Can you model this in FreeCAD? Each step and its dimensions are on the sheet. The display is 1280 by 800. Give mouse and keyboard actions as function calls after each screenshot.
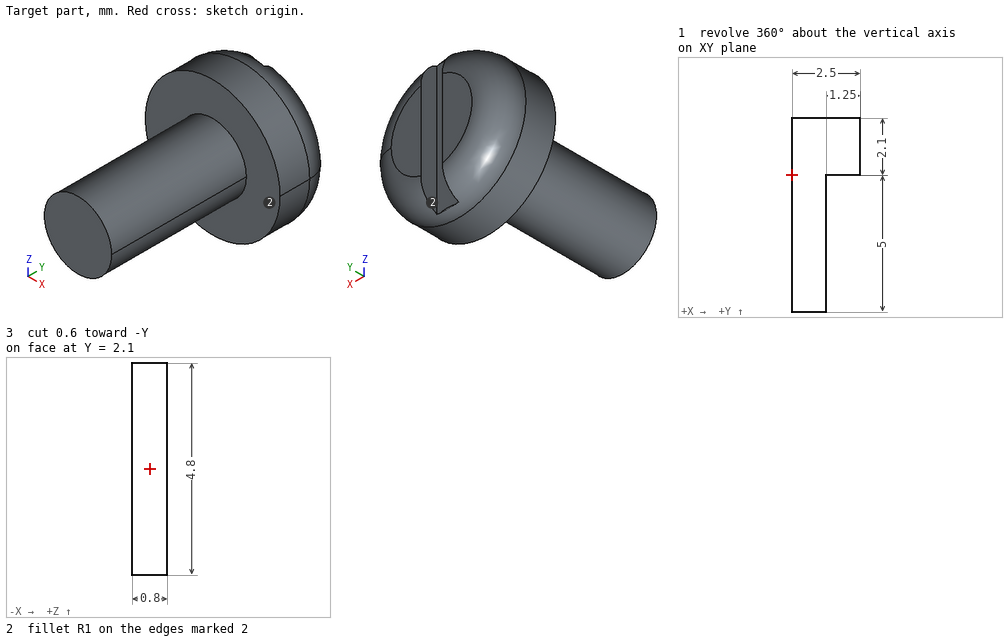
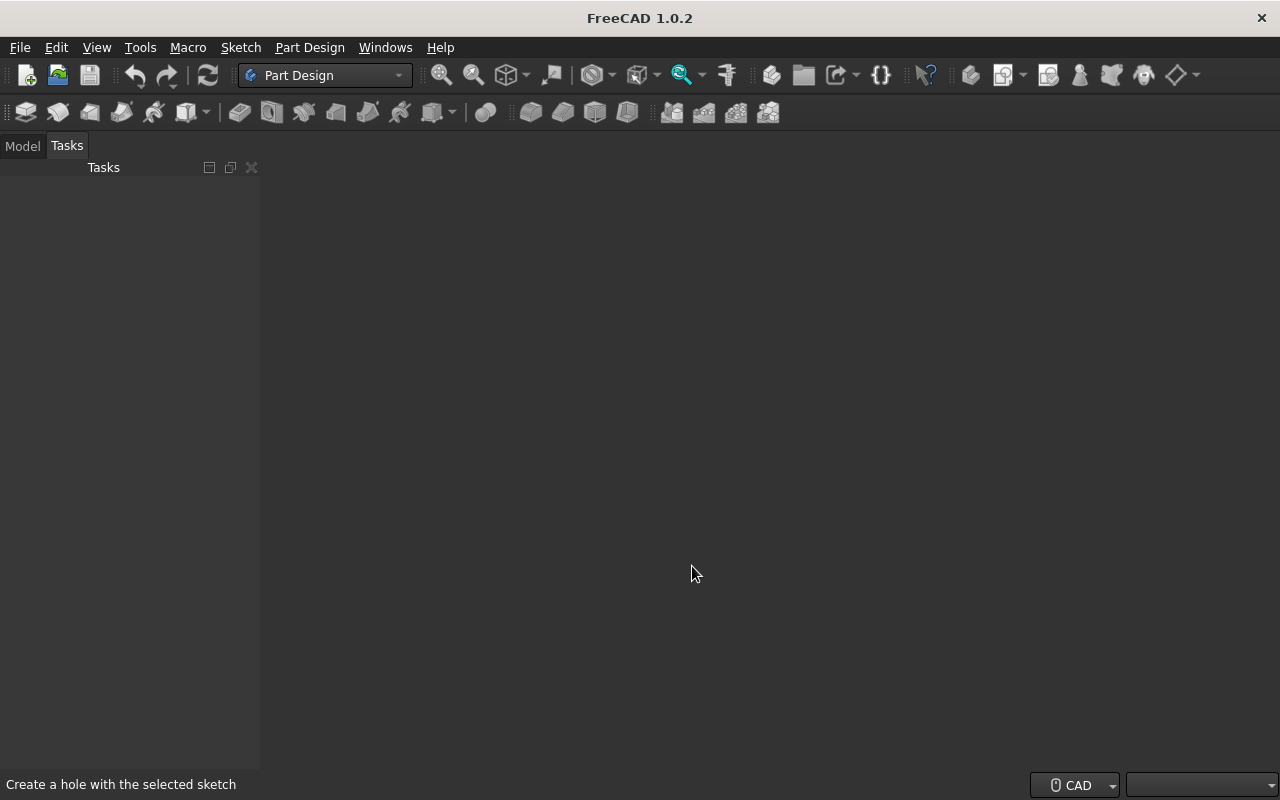
click(26, 76)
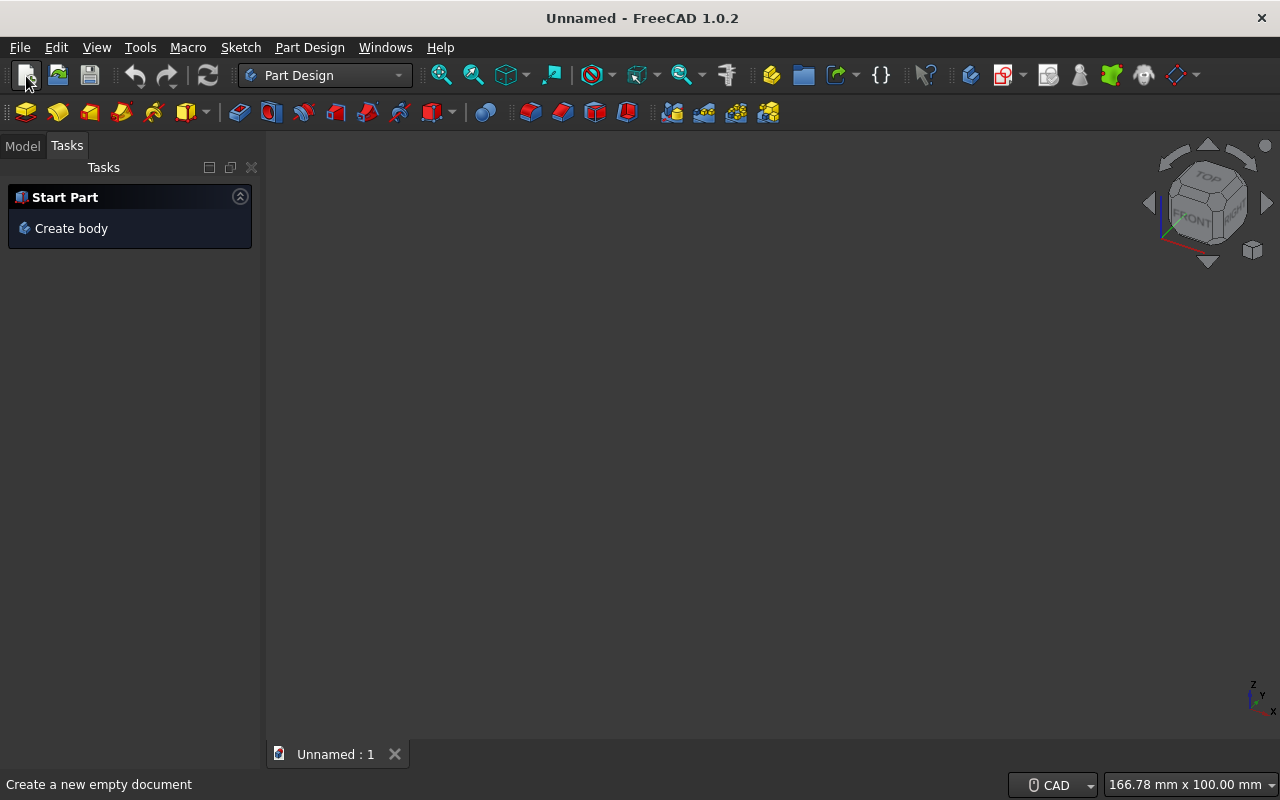
click(1004, 76)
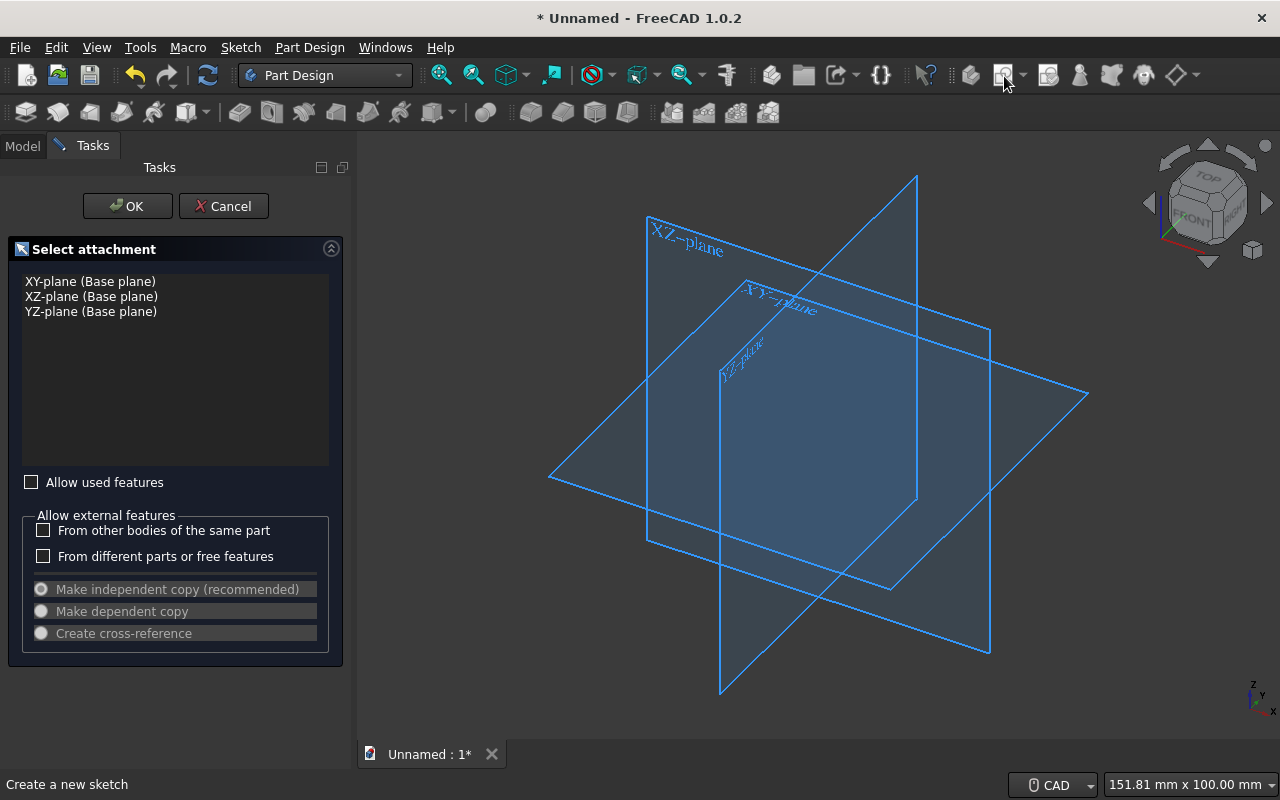
click(82, 282)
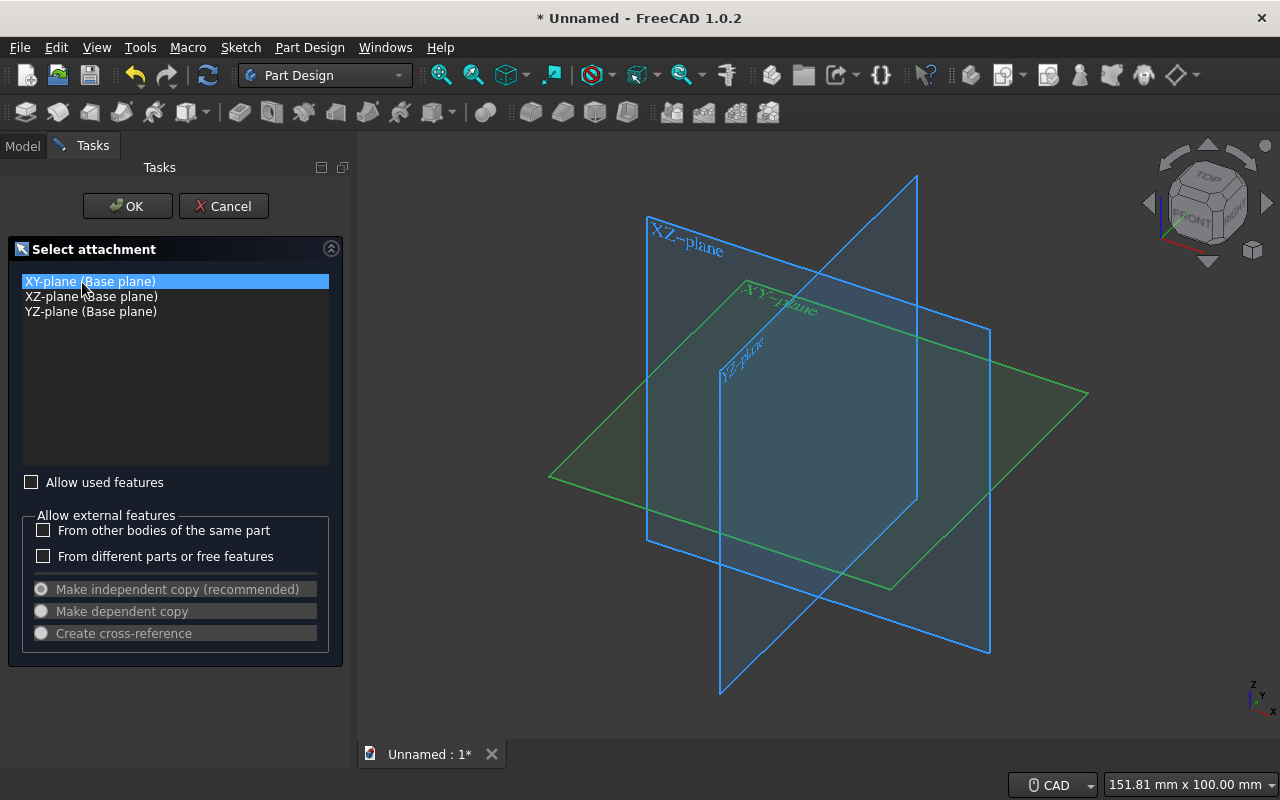
click(128, 206)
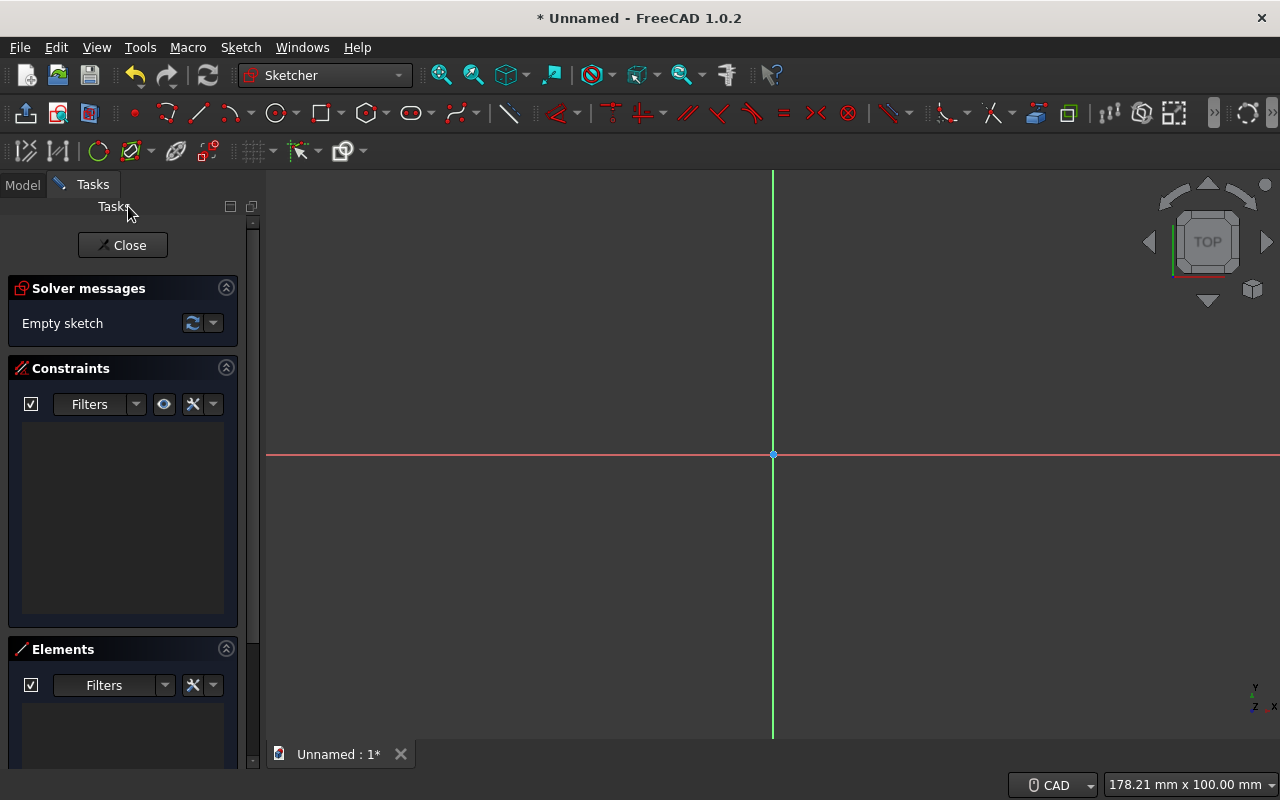
scroll(790, 464, up, 11)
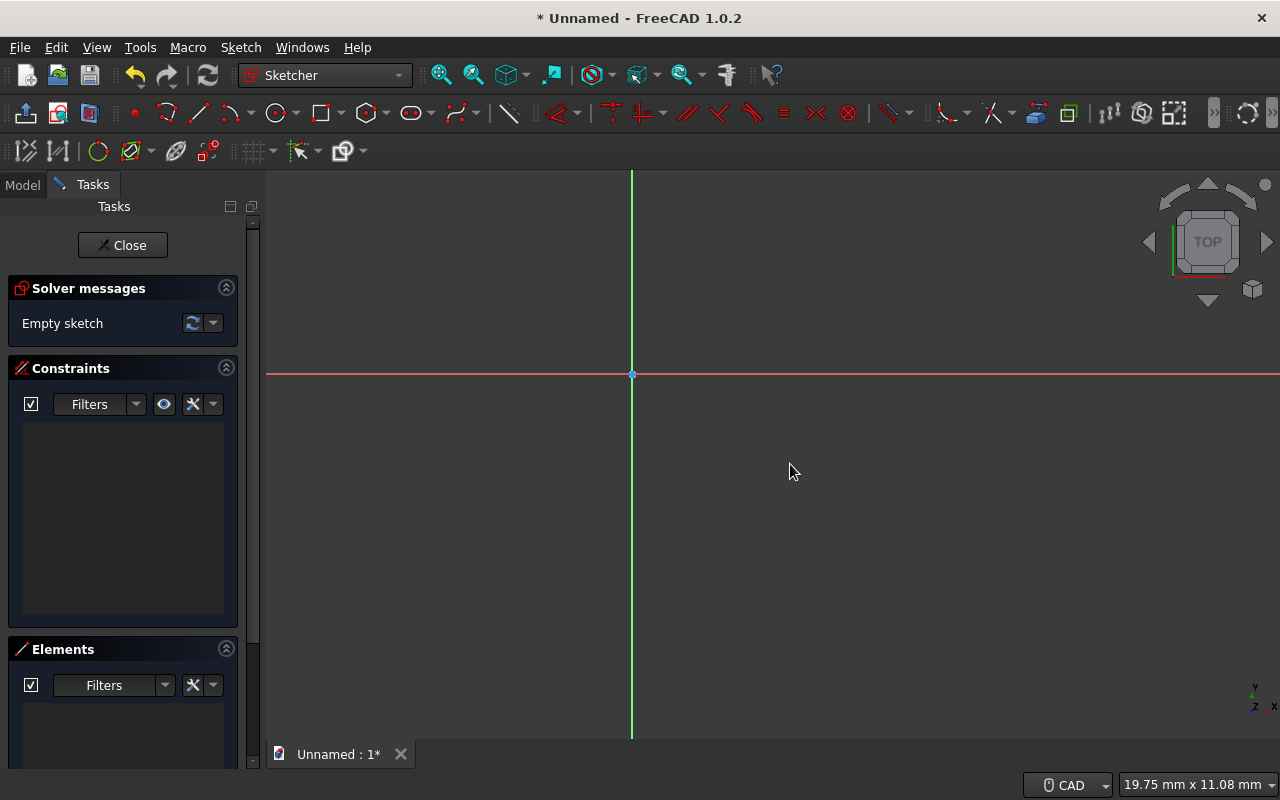
click(168, 114)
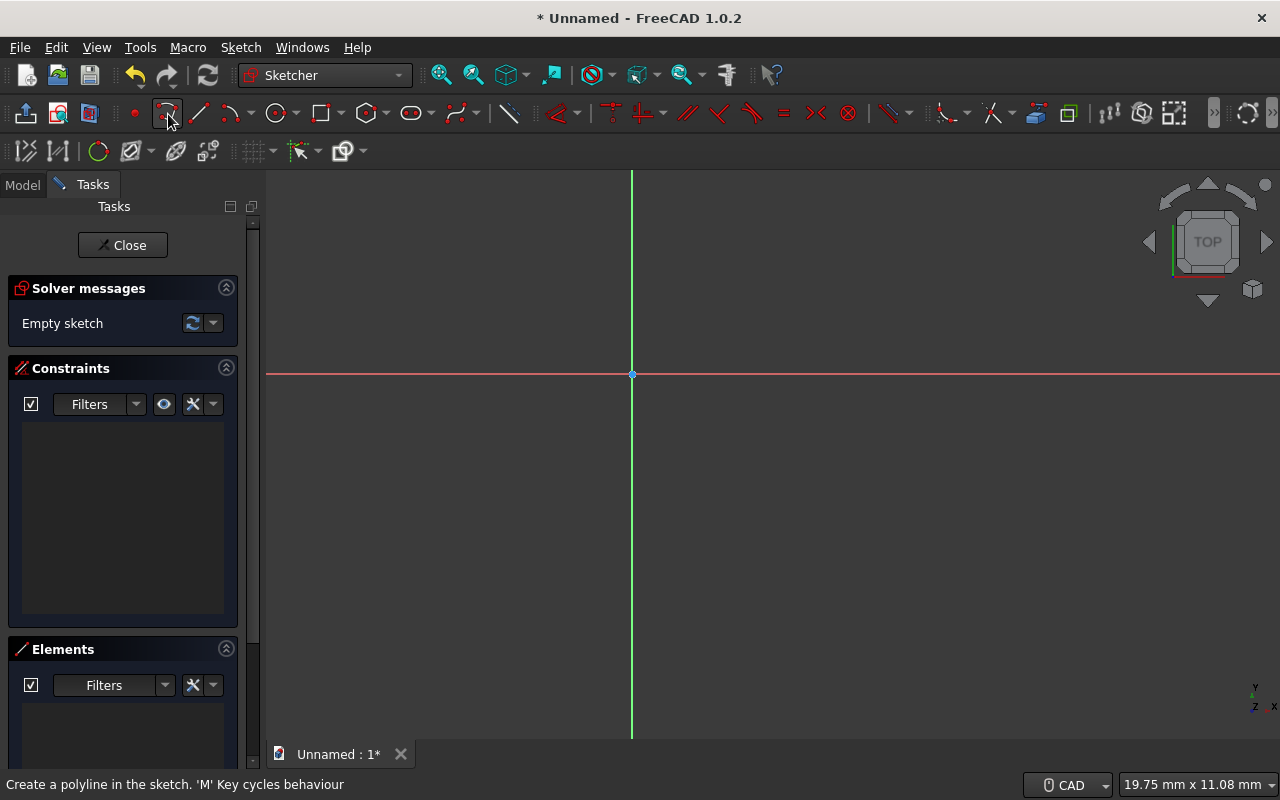
click(697, 374)
click(761, 383)
click(761, 266)
click(632, 266)
click(641, 631)
click(697, 631)
click(697, 374)
key(Escape)
key(Escape)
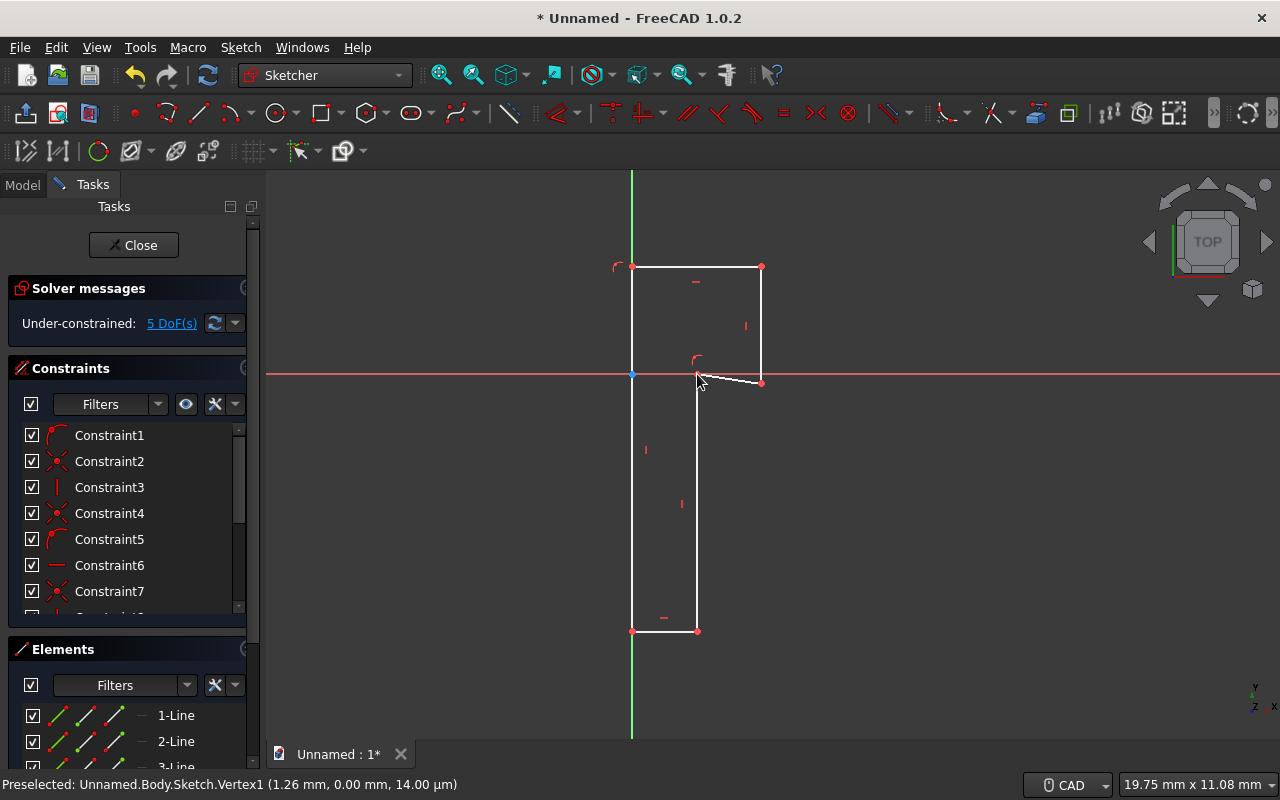
click(716, 377)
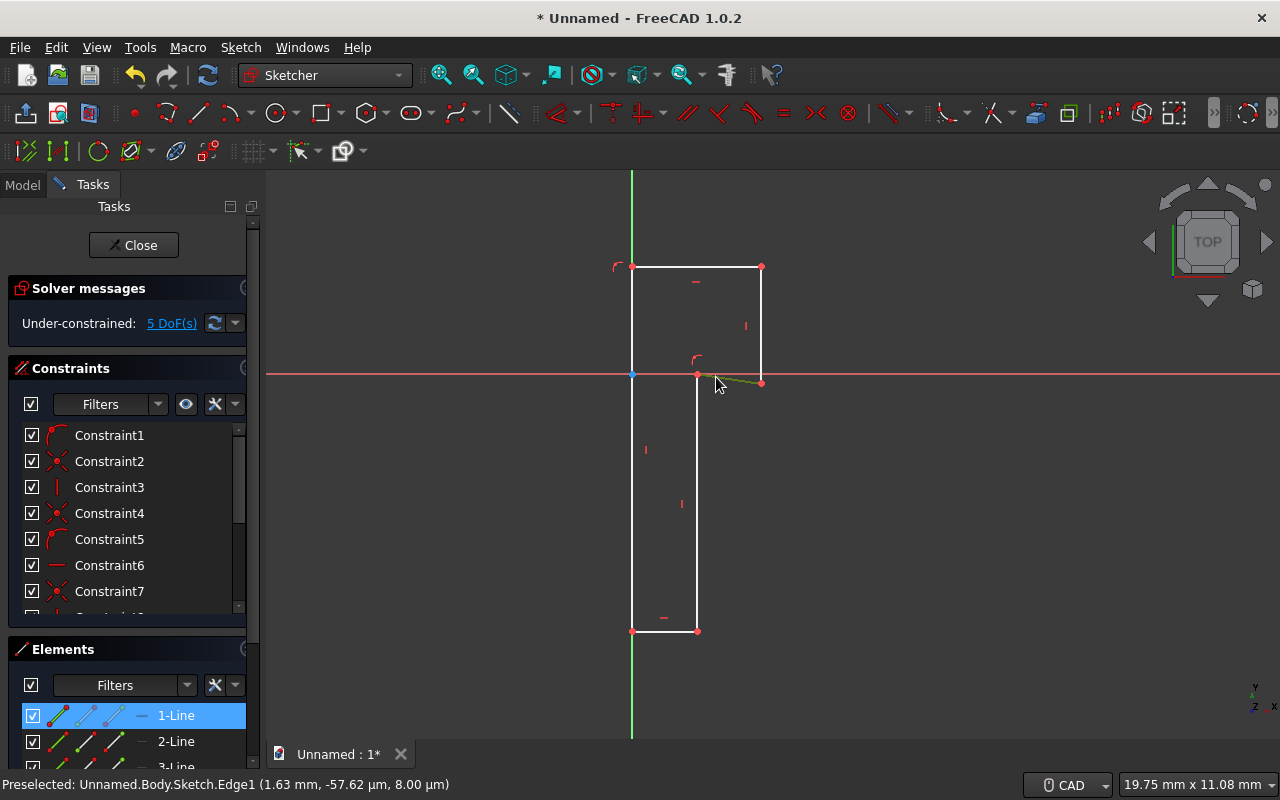
key(h)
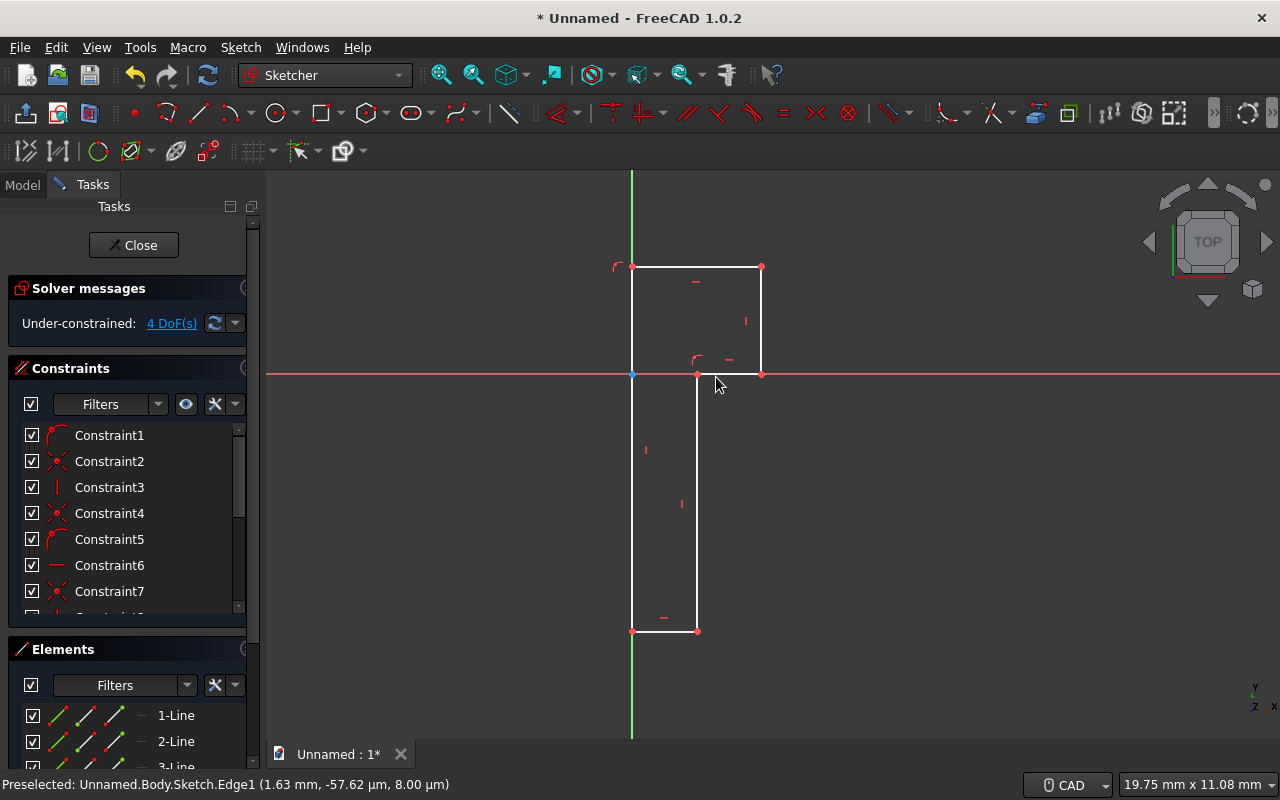
click(556, 114)